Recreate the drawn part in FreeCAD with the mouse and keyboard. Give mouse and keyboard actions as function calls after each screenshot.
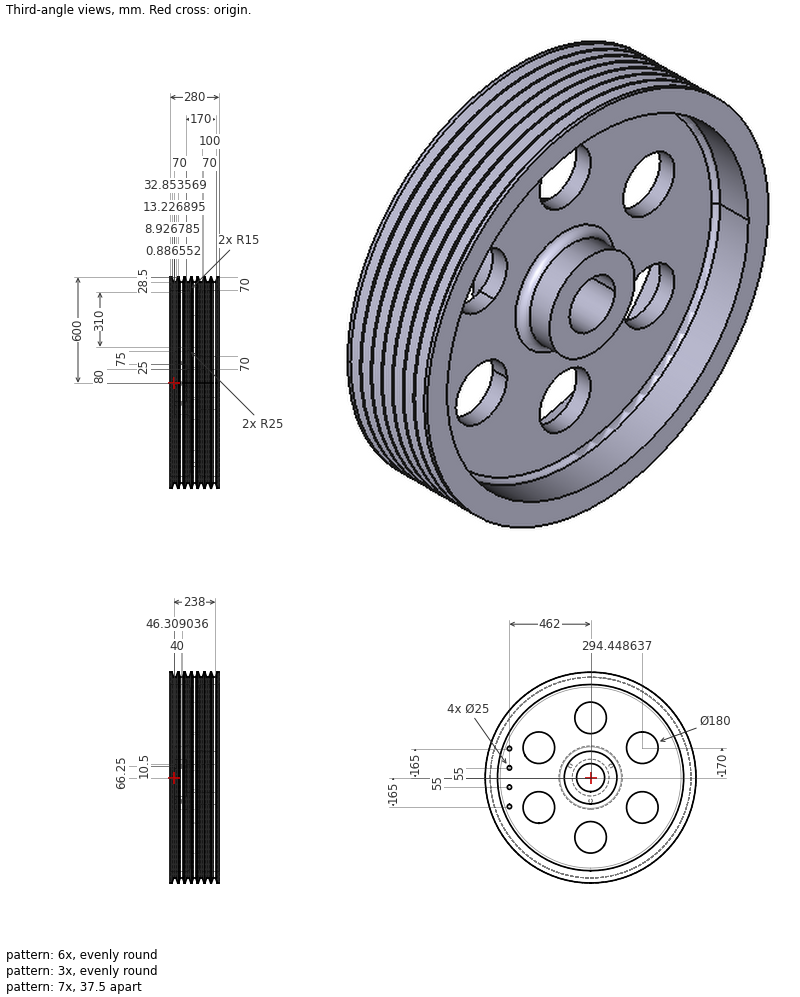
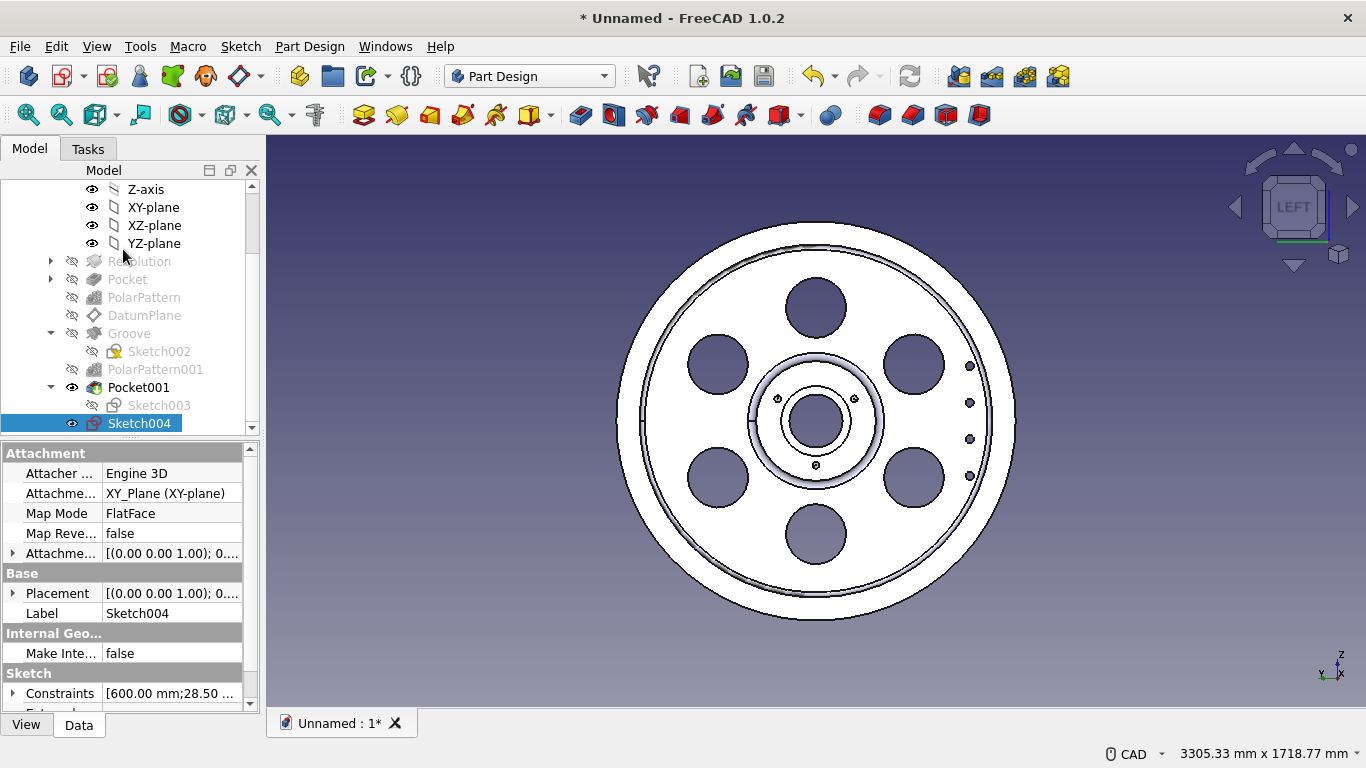
click(647, 116)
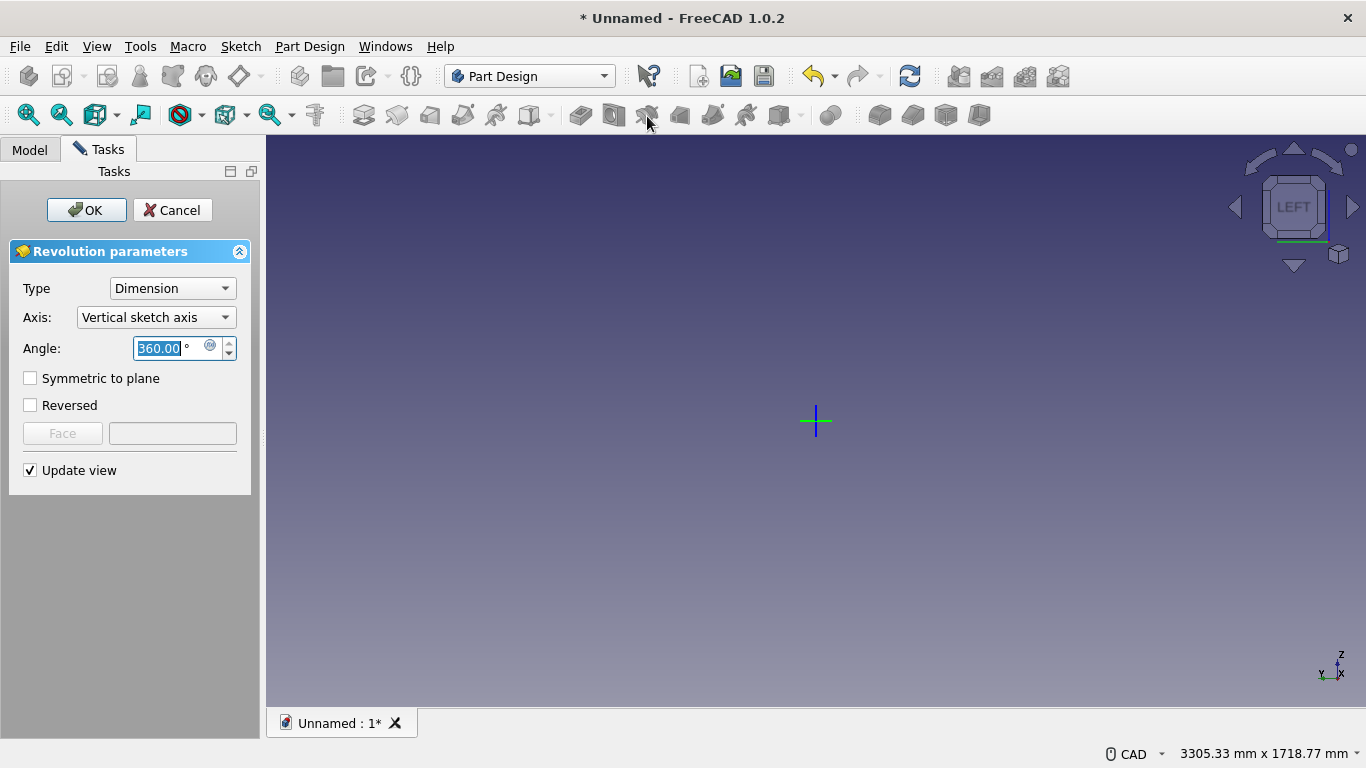
click(157, 318)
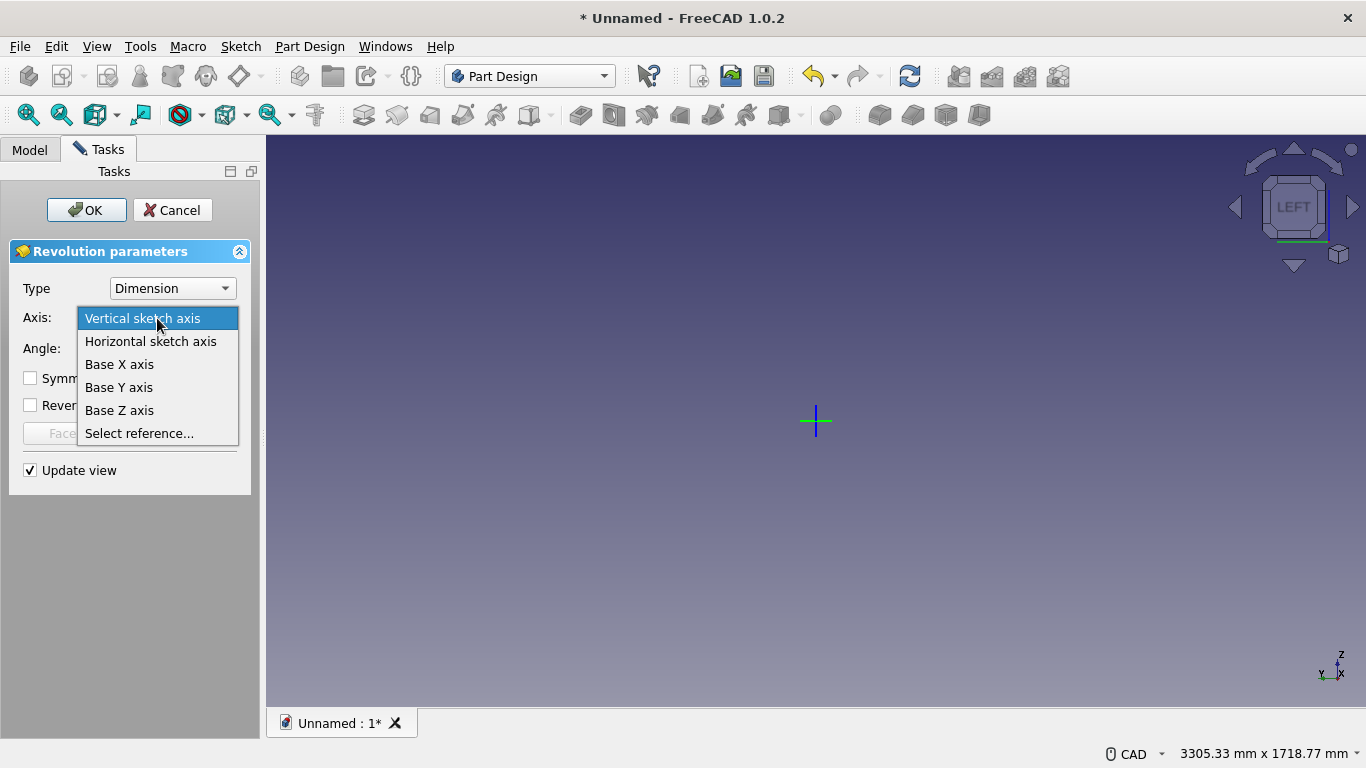
click(156, 342)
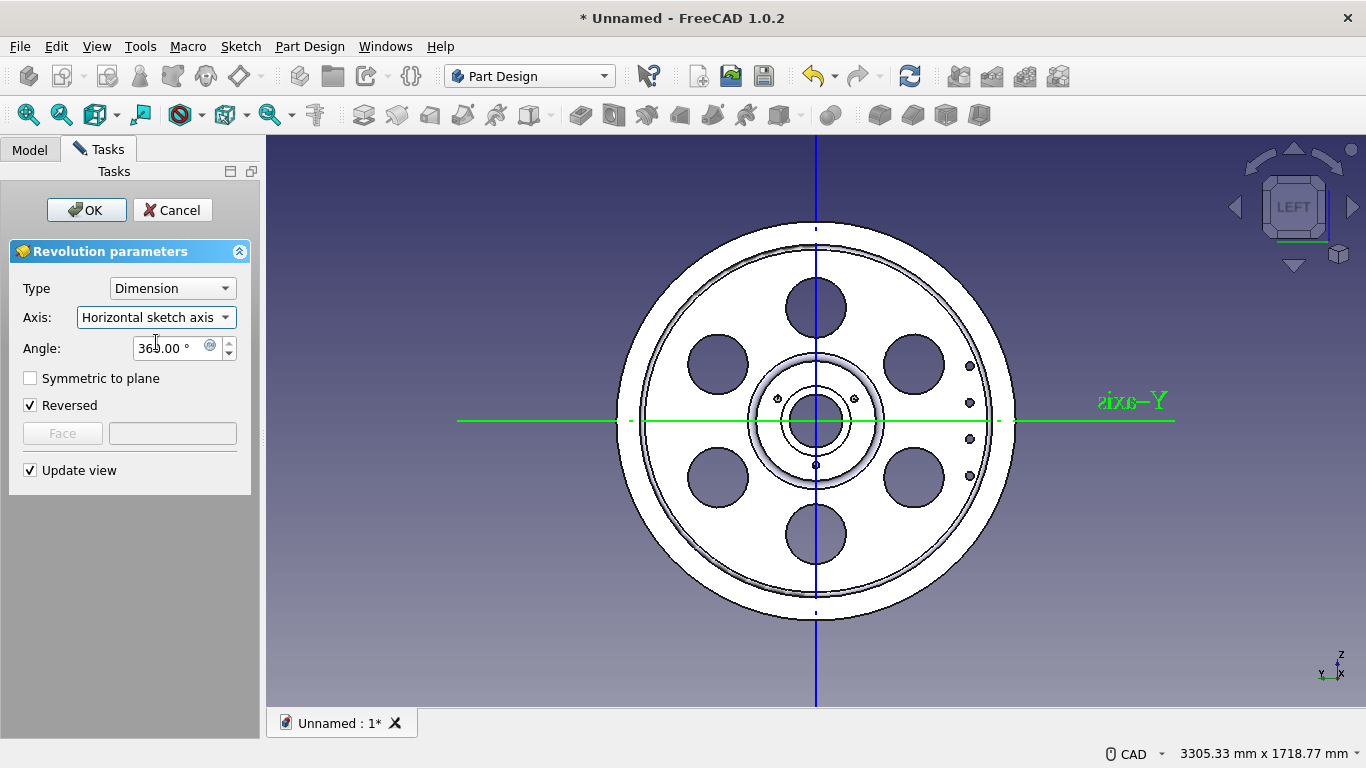
click(87, 210)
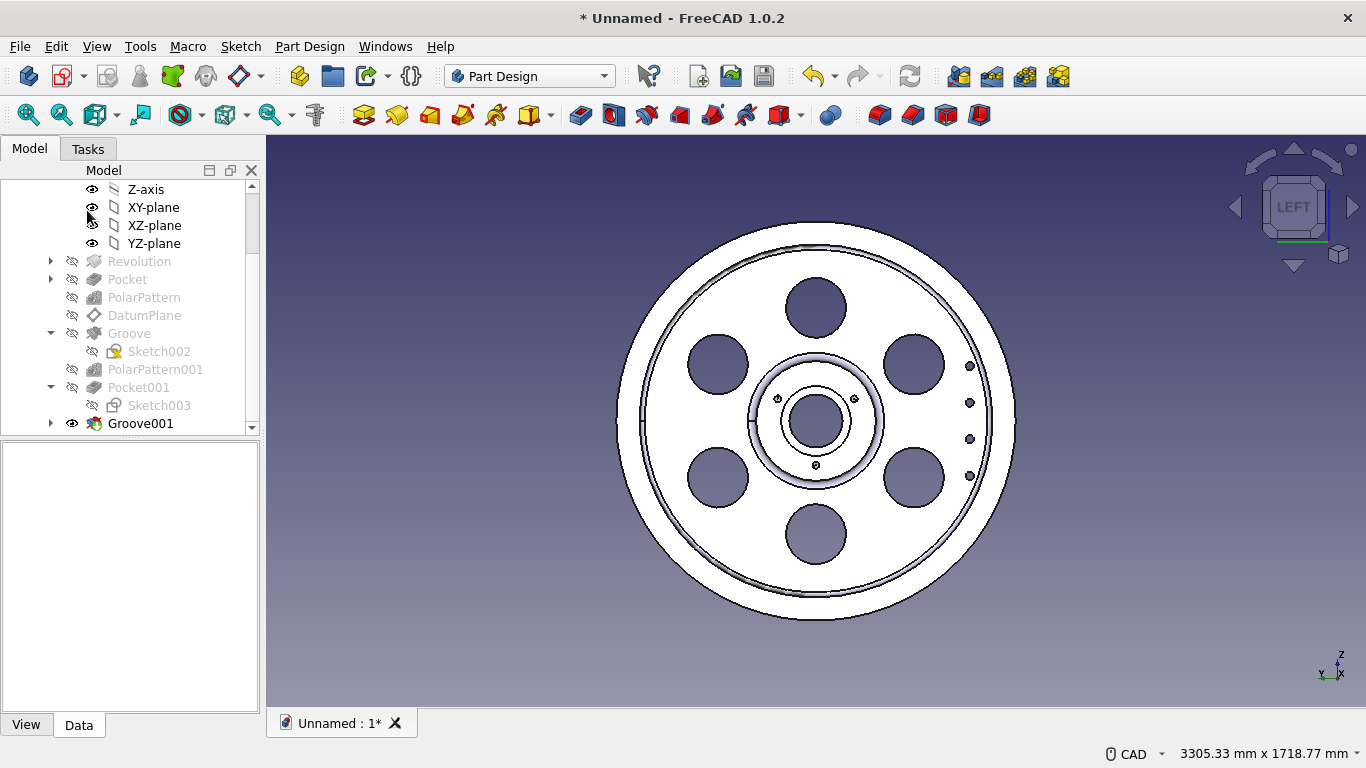
click(117, 423)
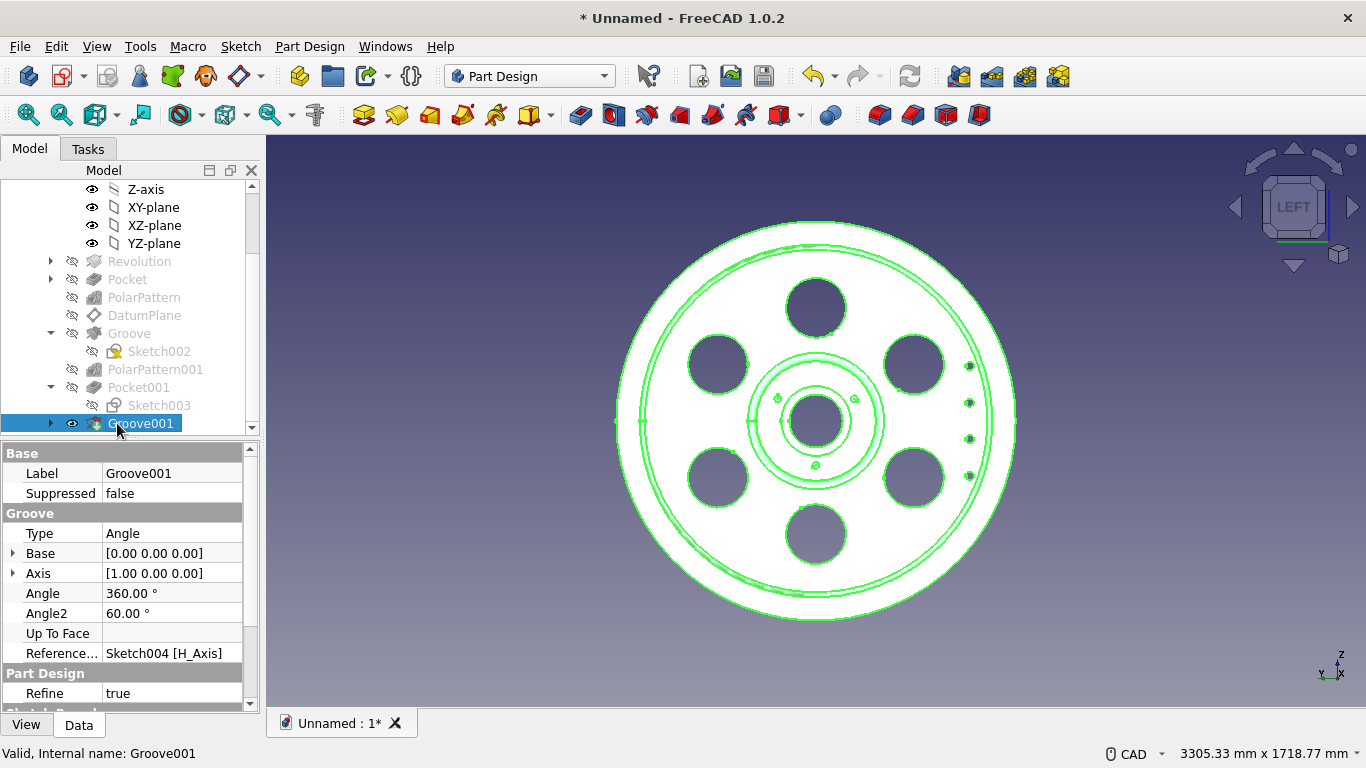
click(992, 76)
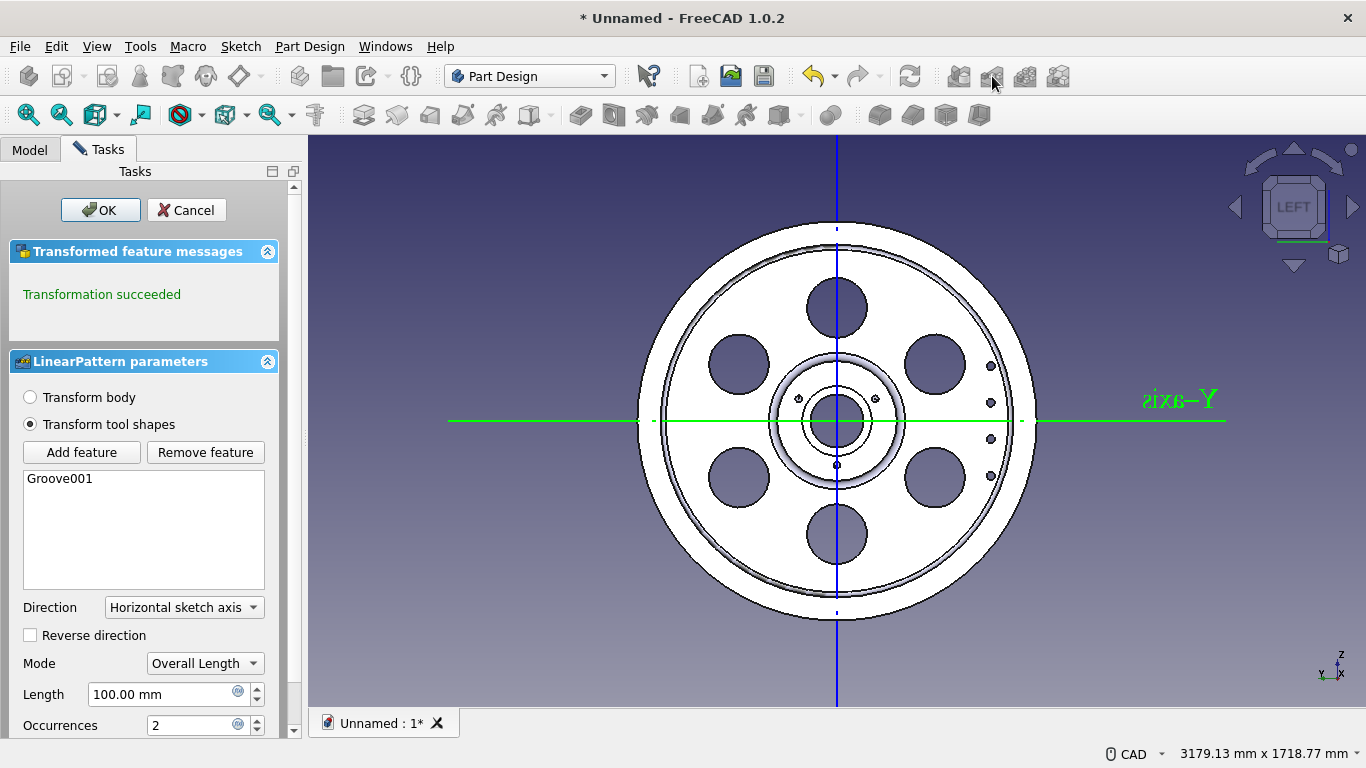
click(185, 608)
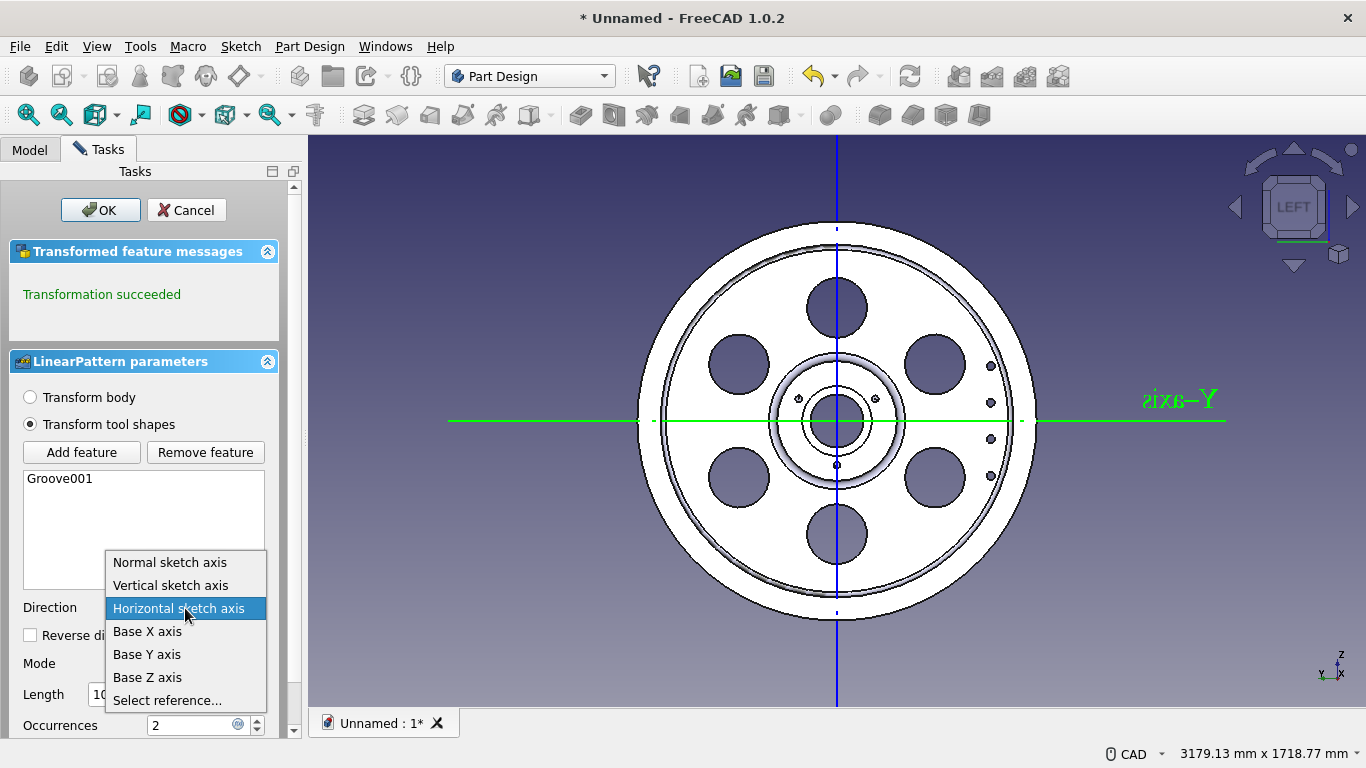
click(184, 632)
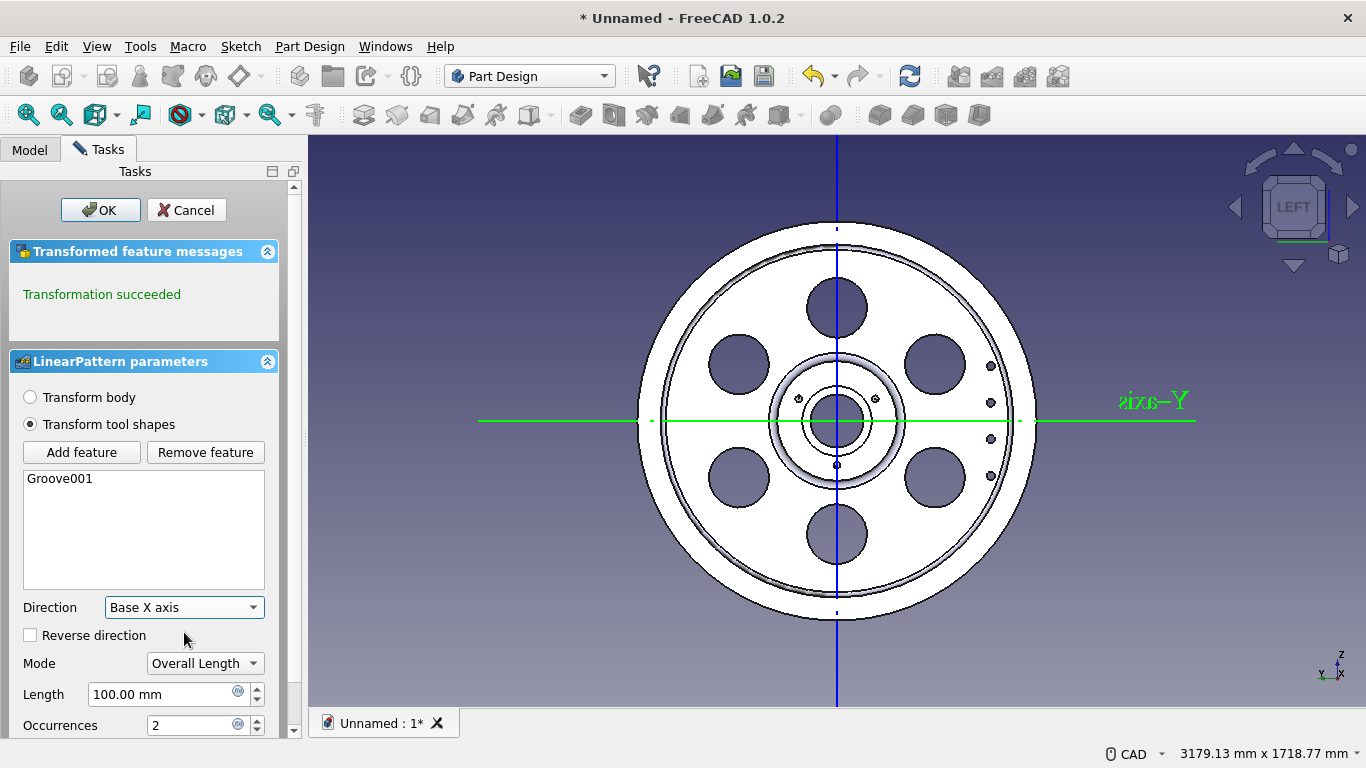
click(206, 664)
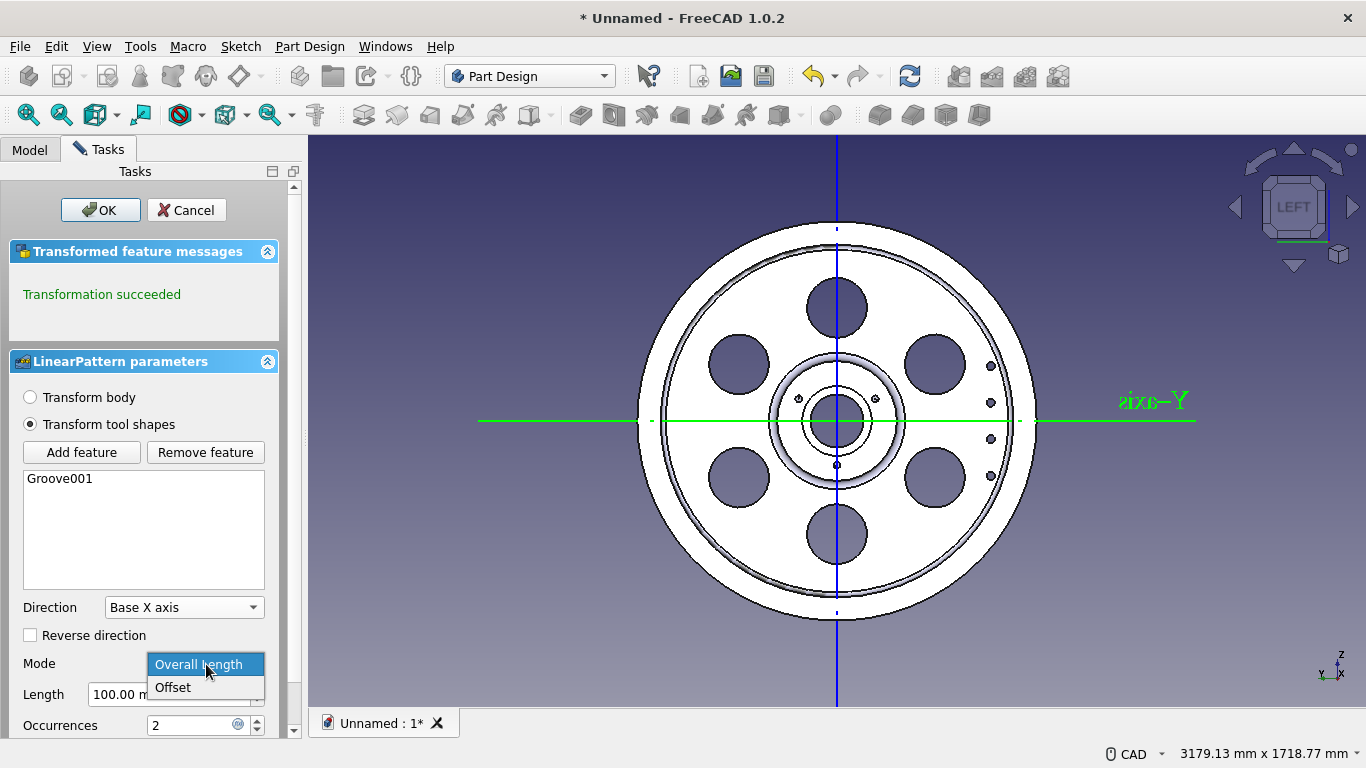
click(204, 688)